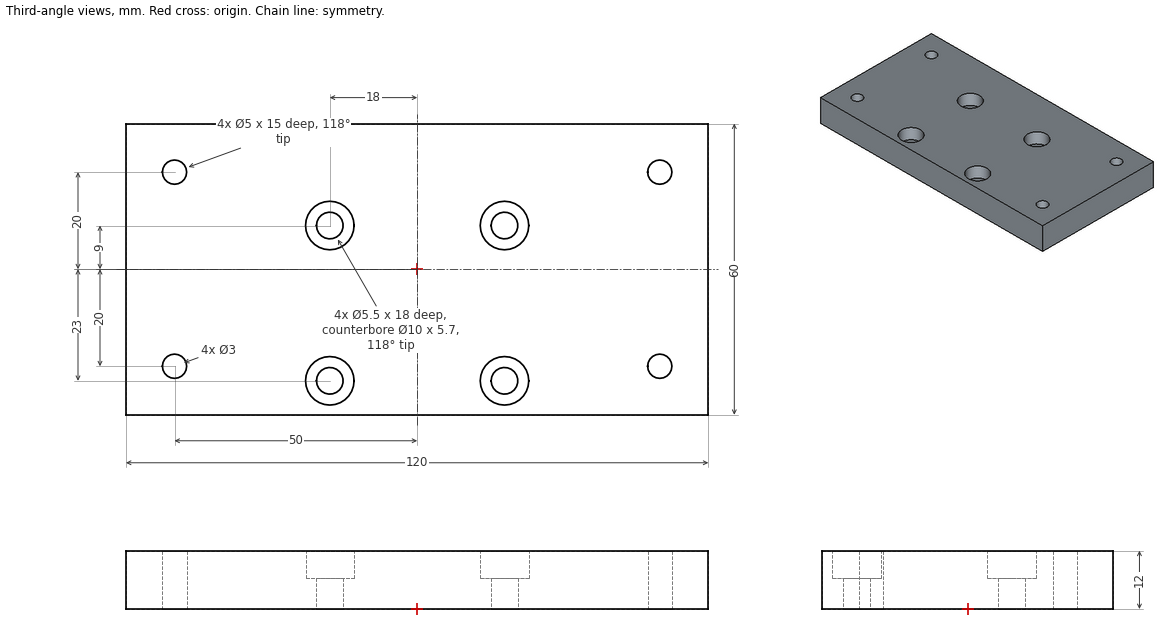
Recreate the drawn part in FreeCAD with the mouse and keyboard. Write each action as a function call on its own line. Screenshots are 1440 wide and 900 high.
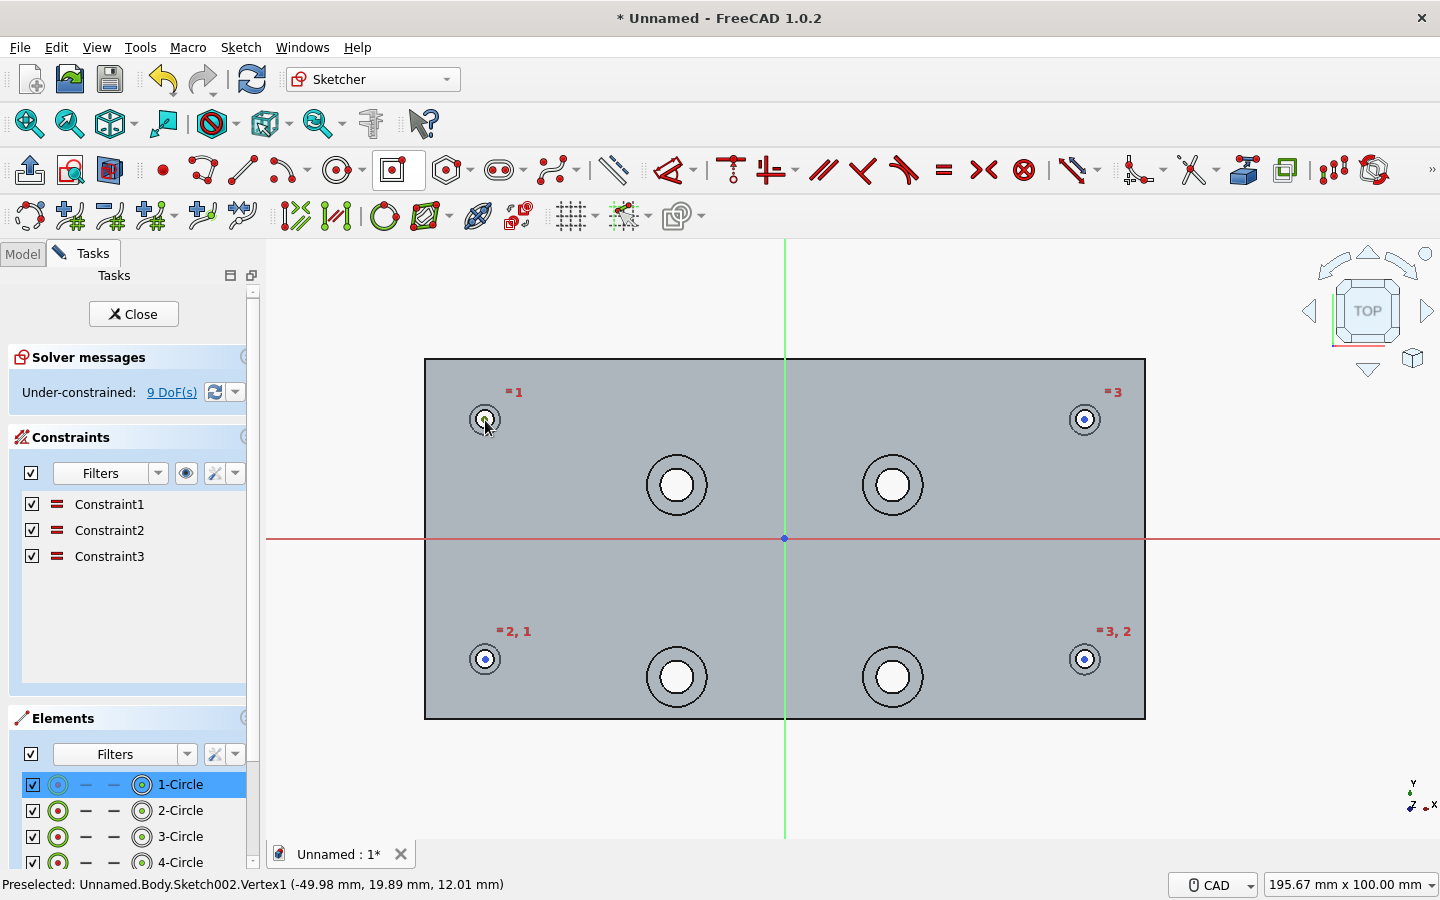
click(485, 659)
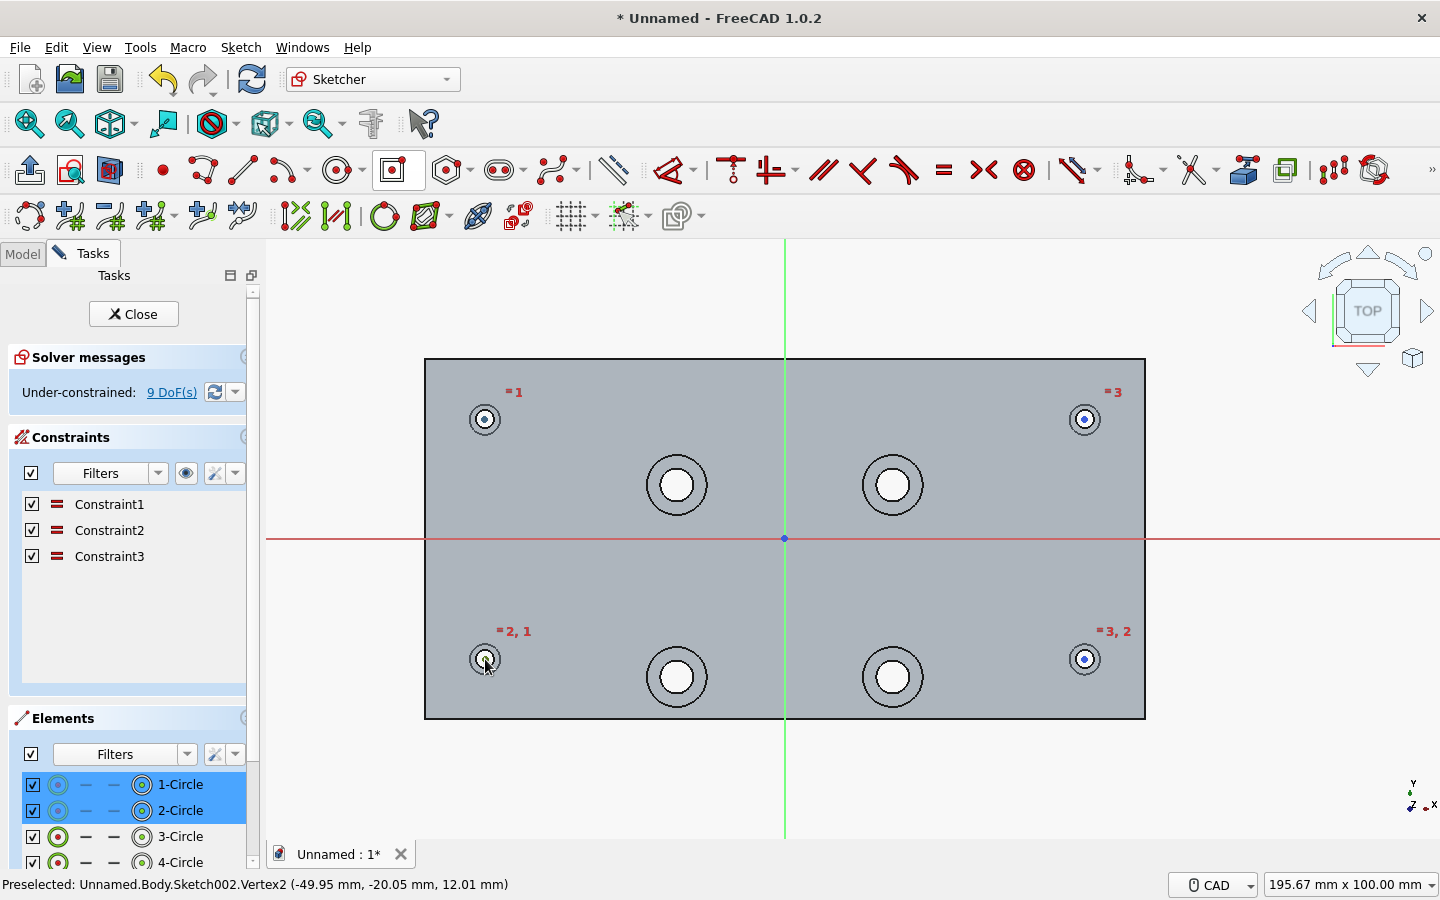
click(364, 539)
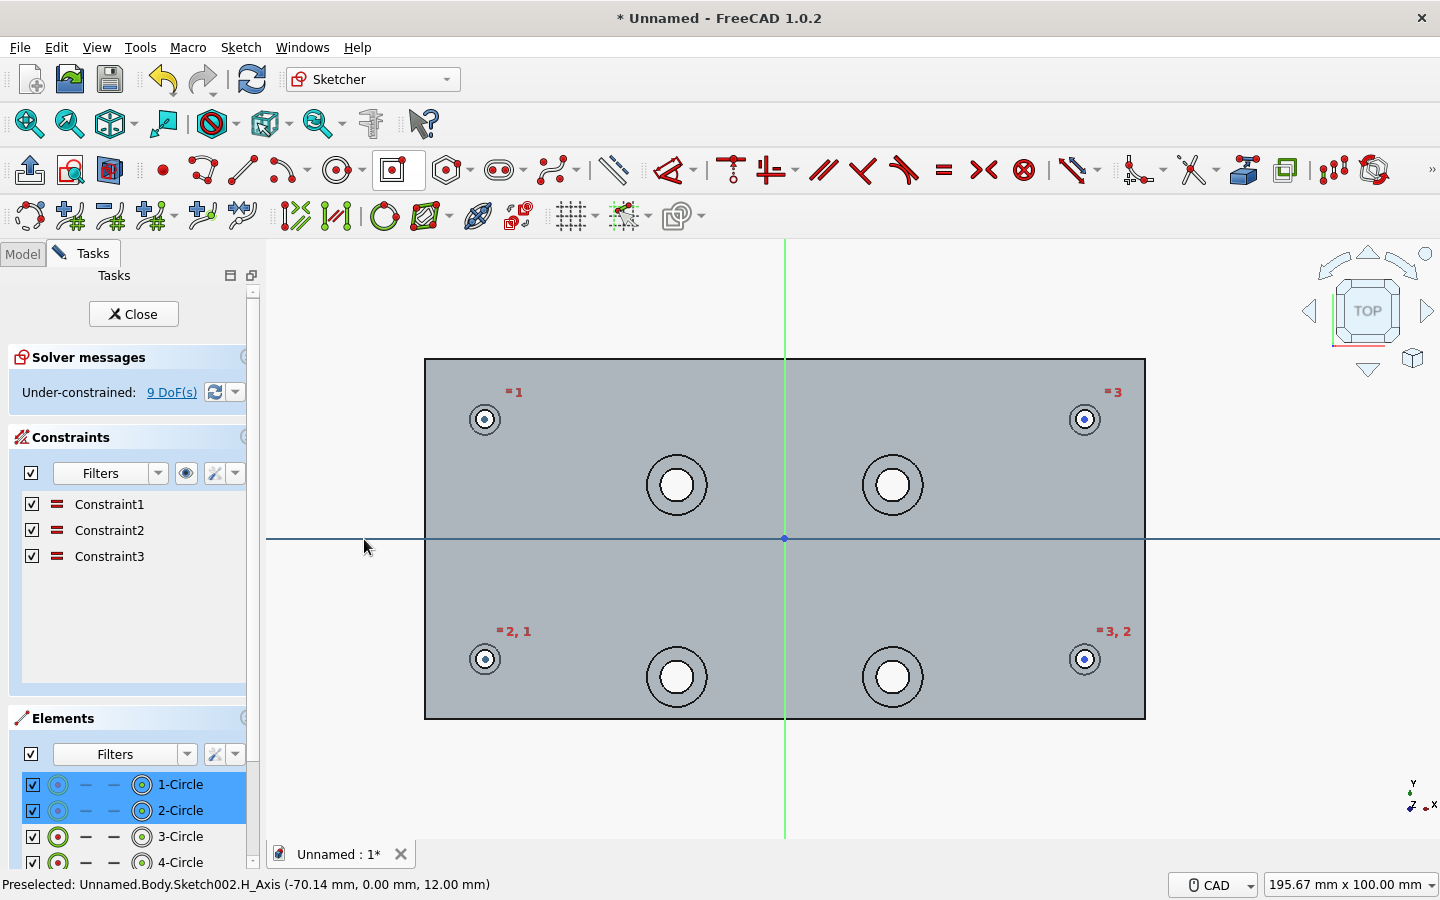
click(984, 170)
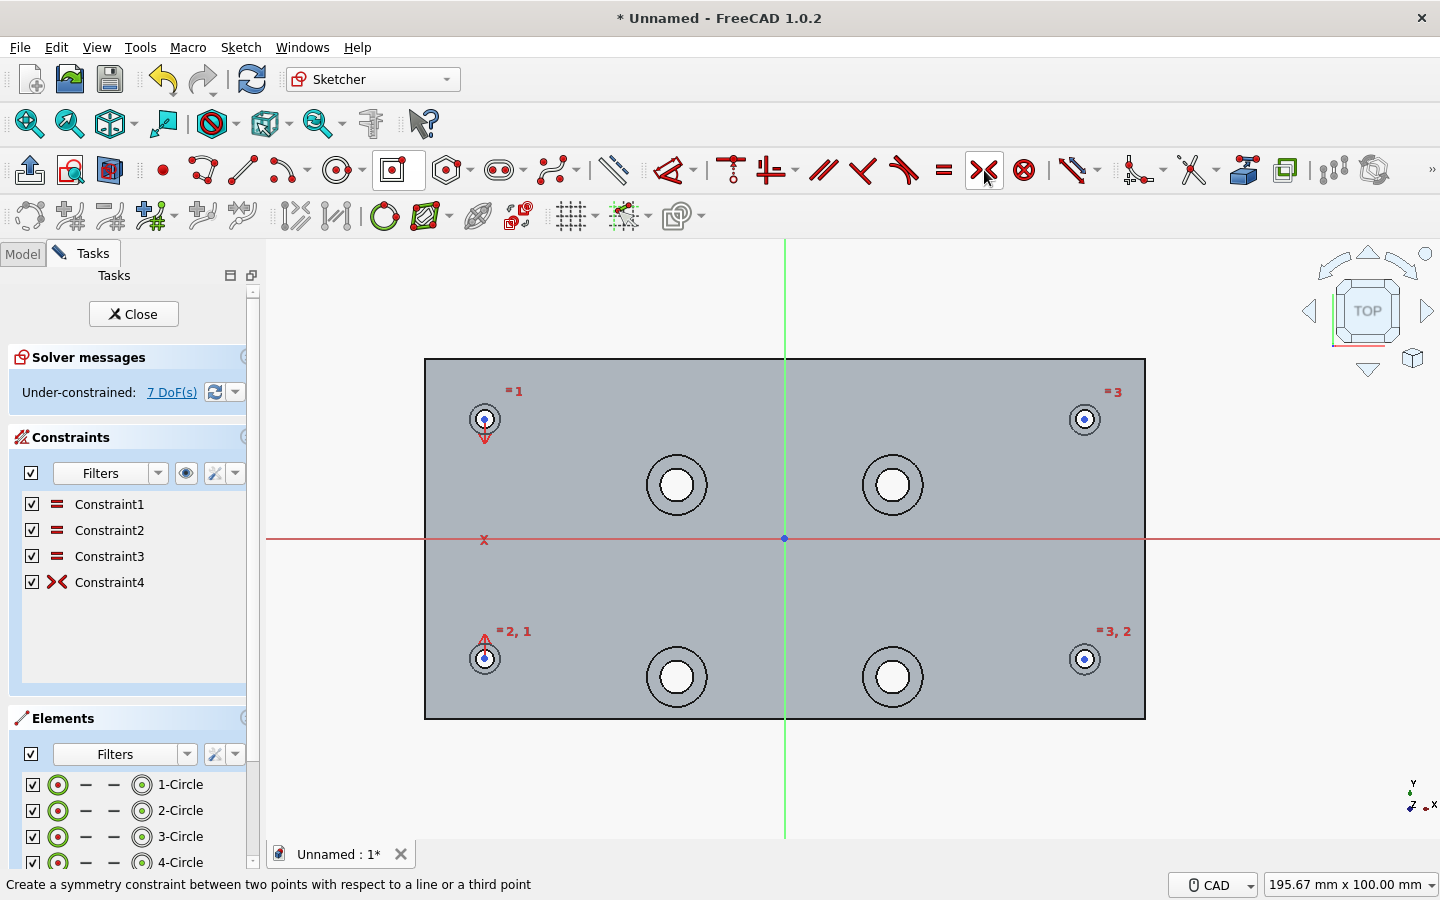
click(485, 659)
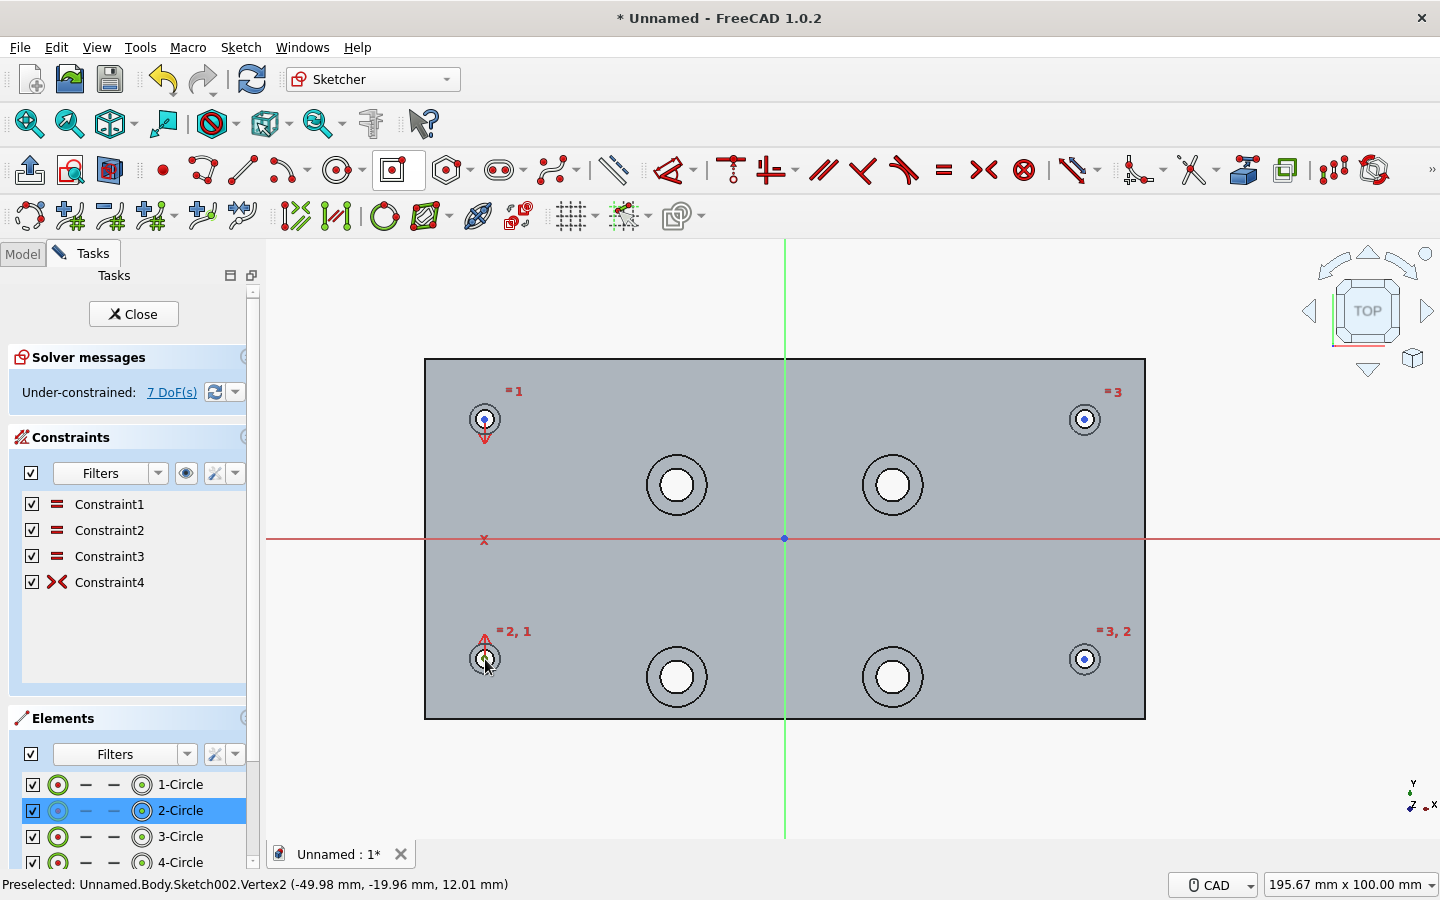
click(1085, 659)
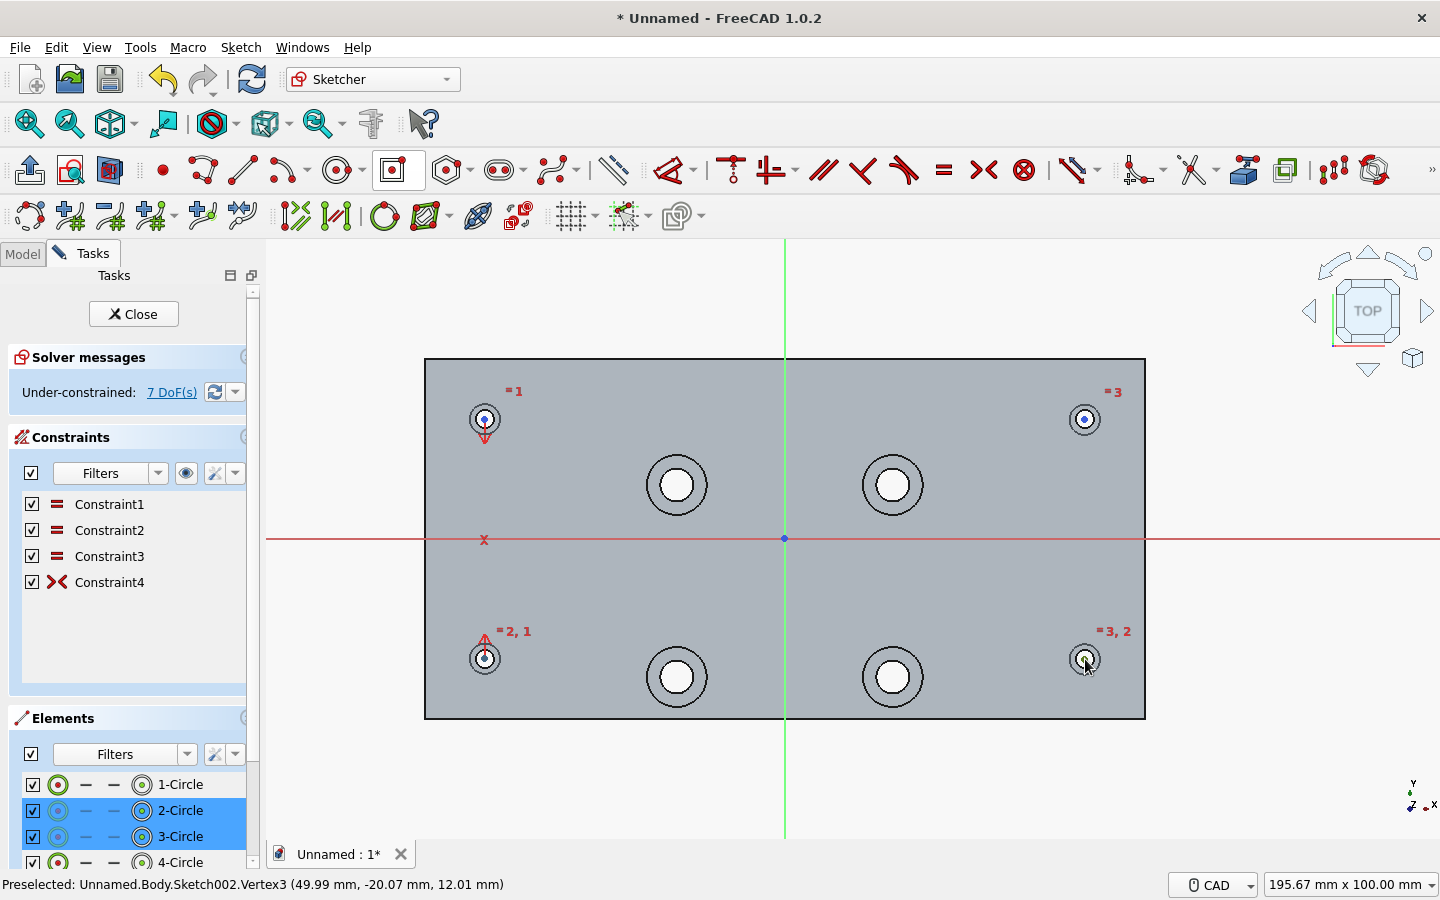
click(785, 772)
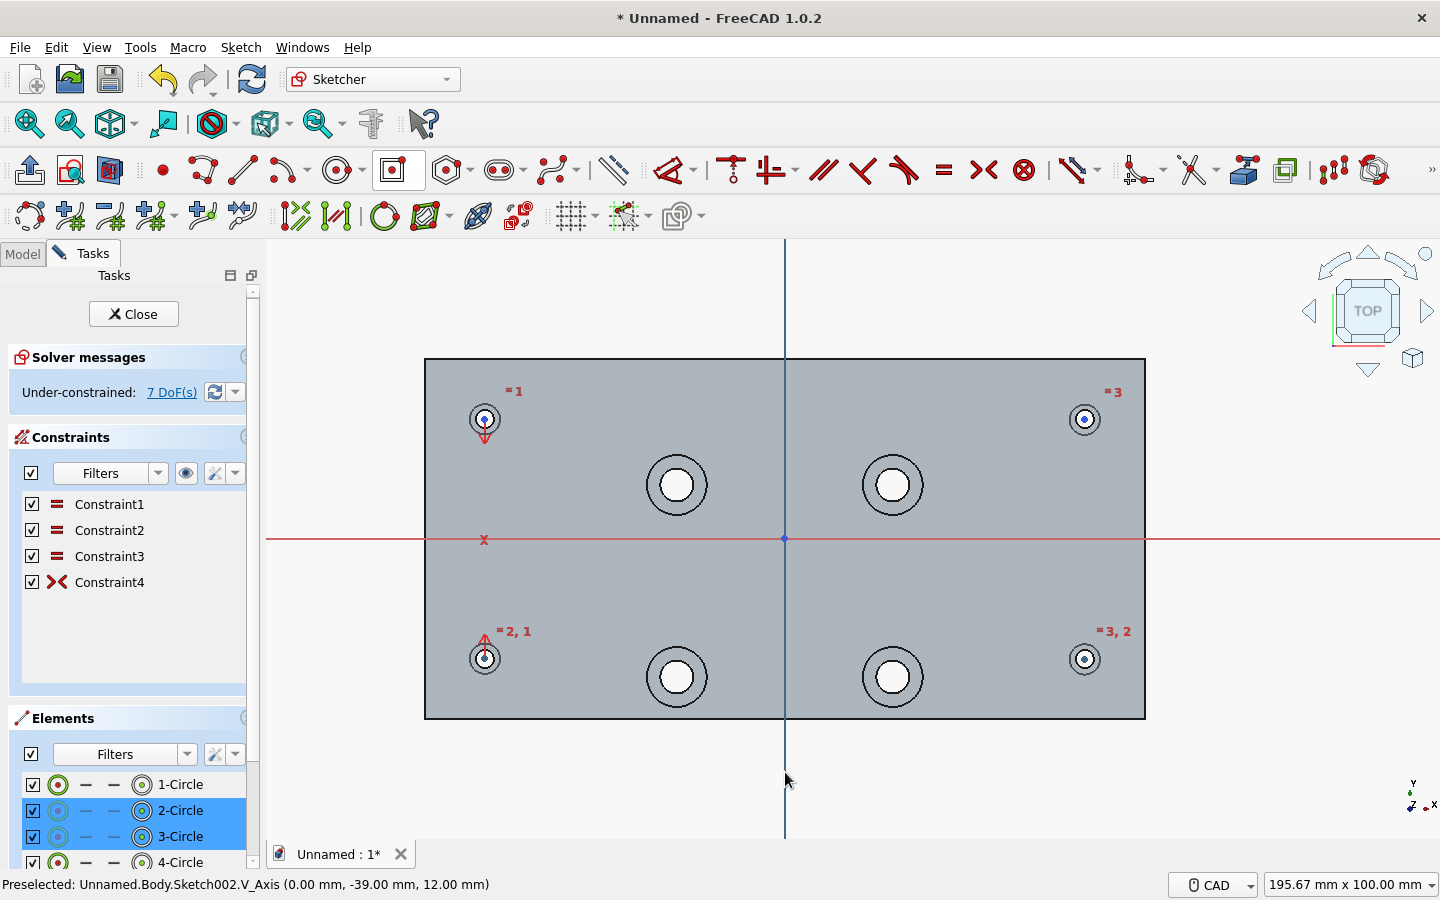
click(984, 170)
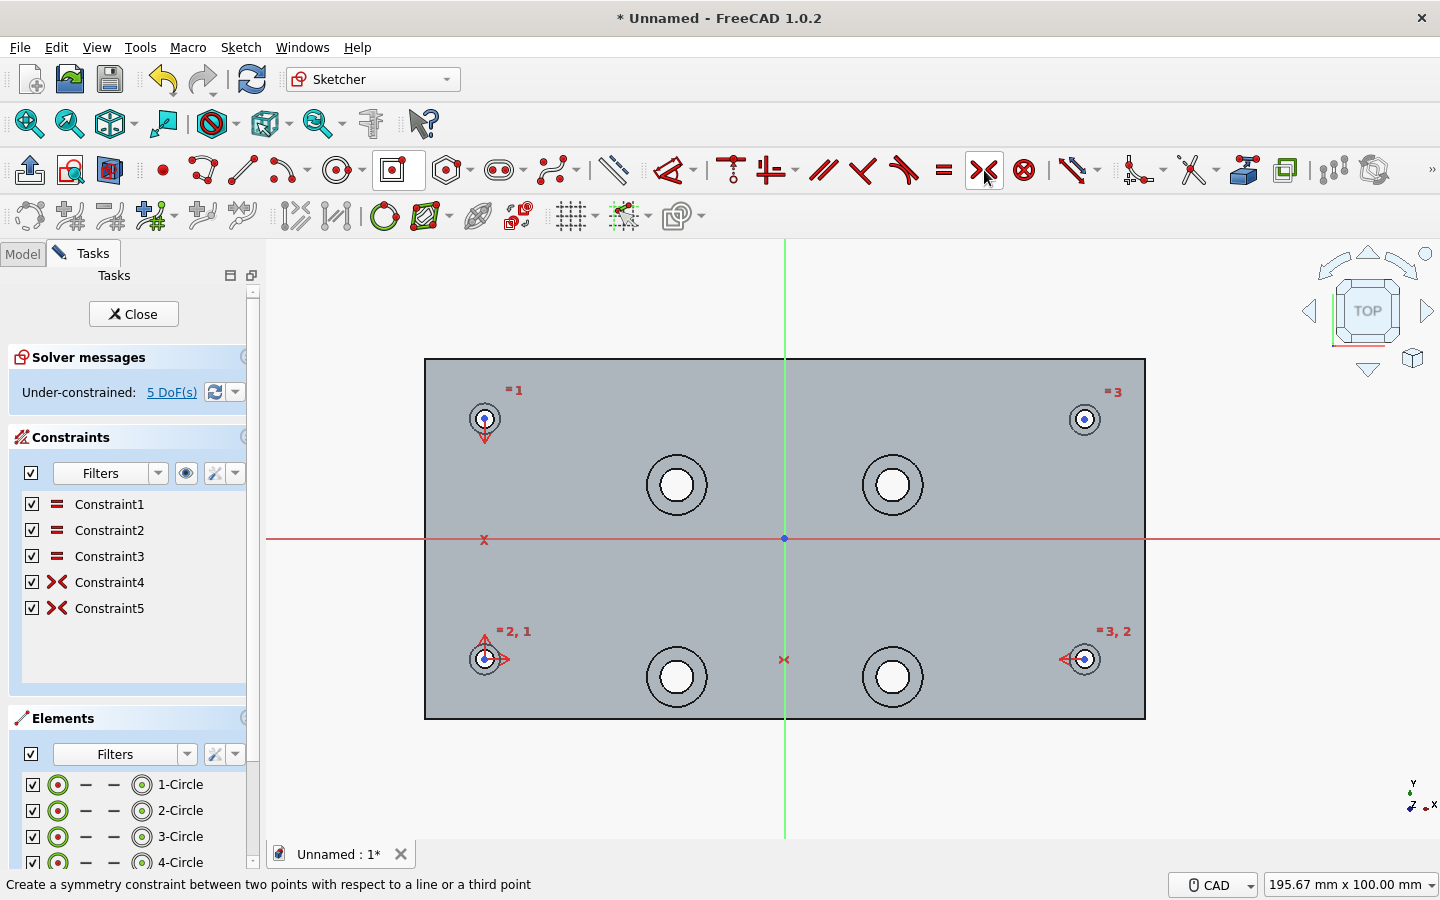
click(485, 419)